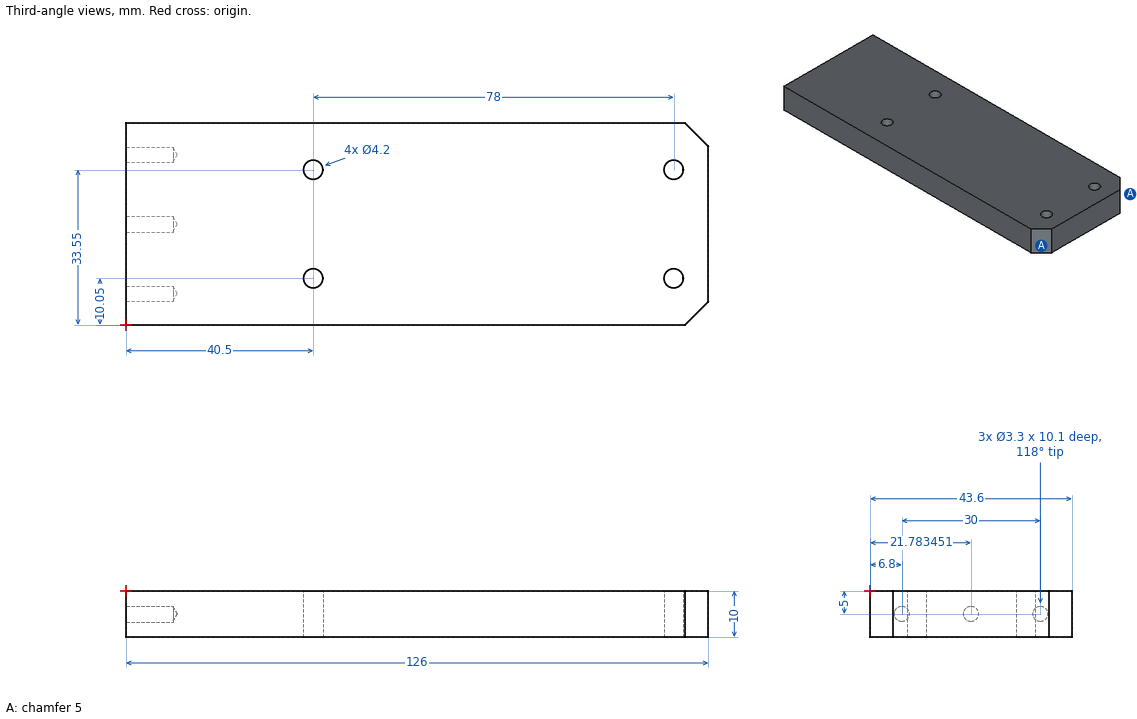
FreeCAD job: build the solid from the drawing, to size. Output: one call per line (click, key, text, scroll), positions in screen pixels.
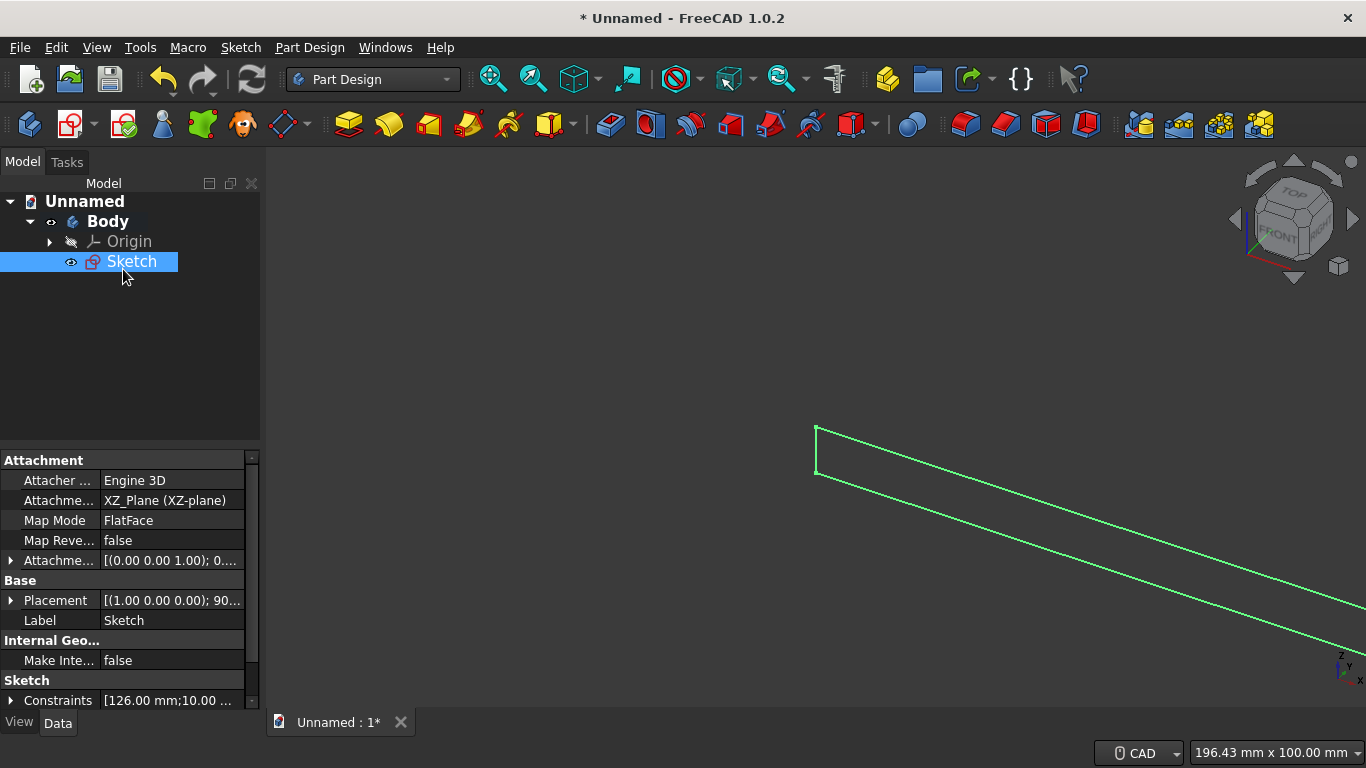
click(350, 124)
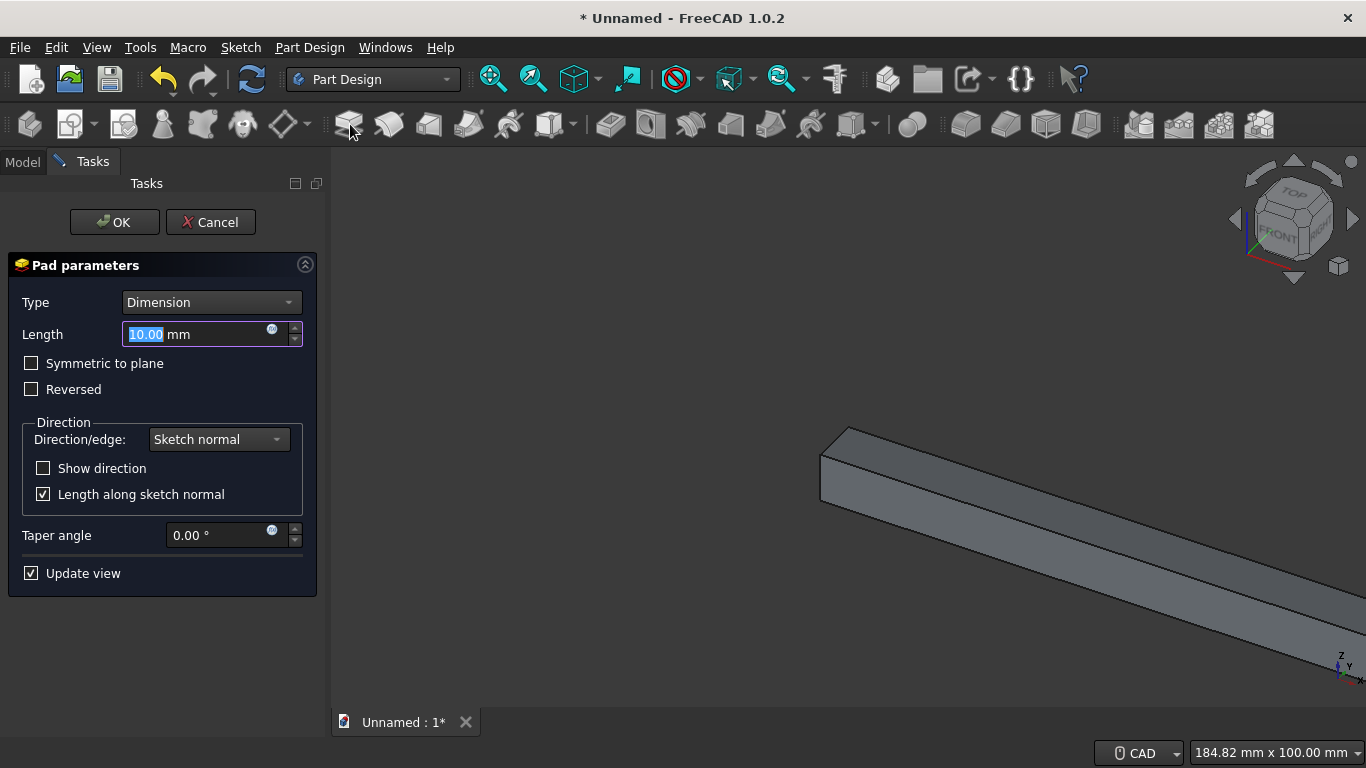
text(43.6)
key(Tab)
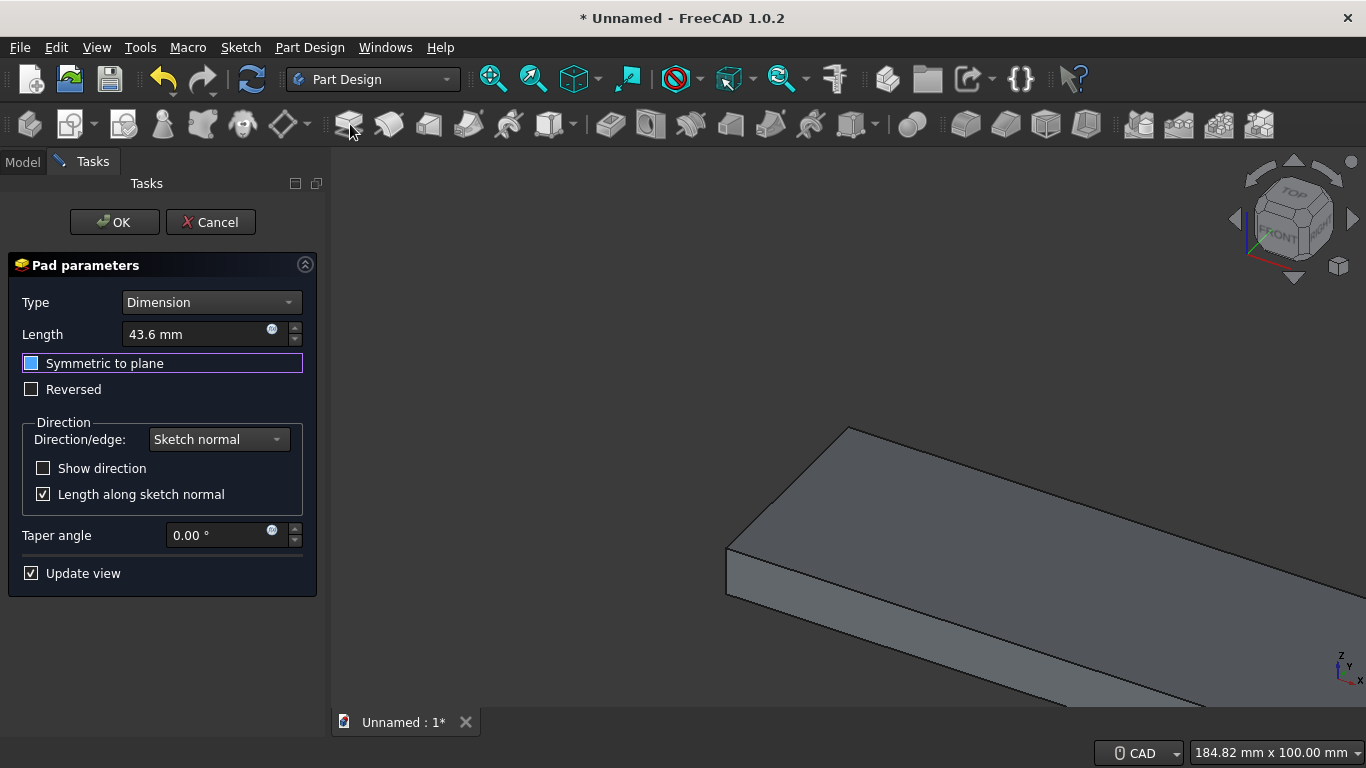
click(30, 389)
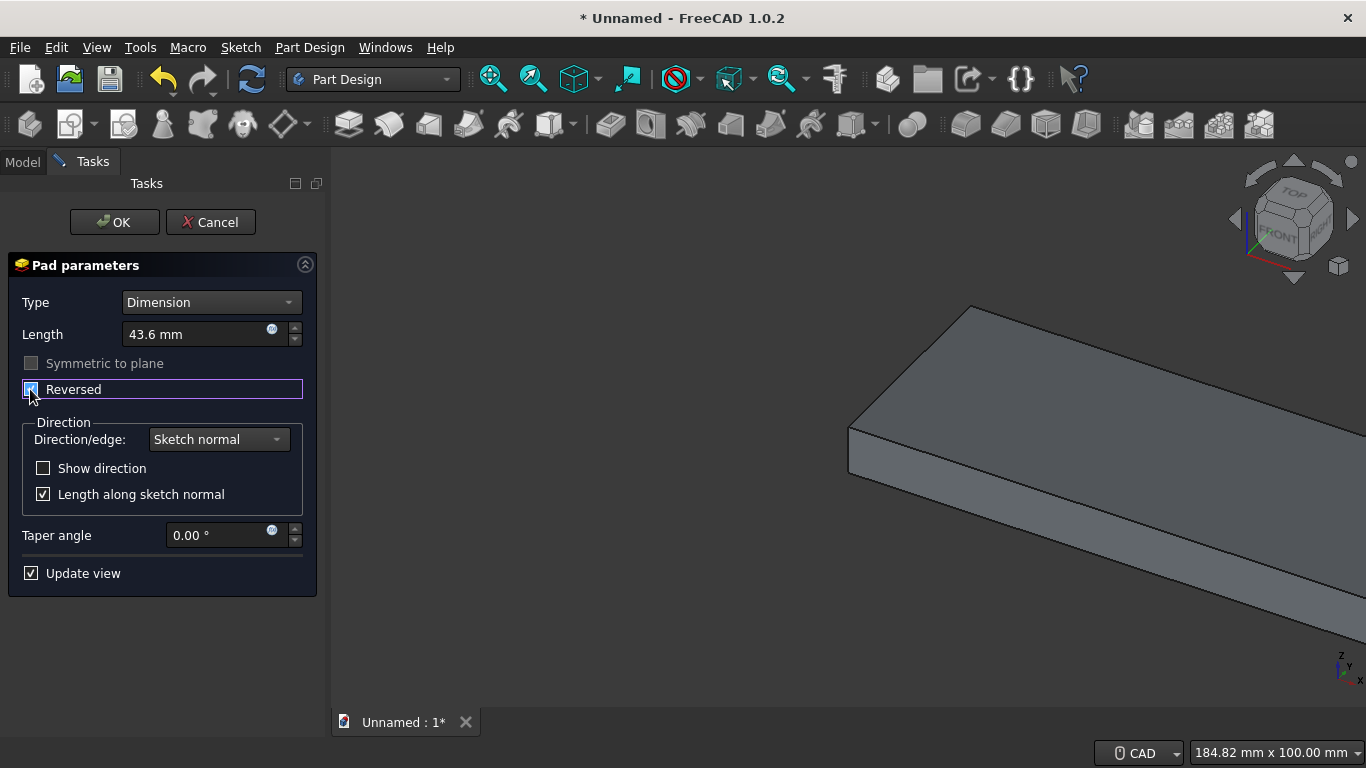
click(115, 222)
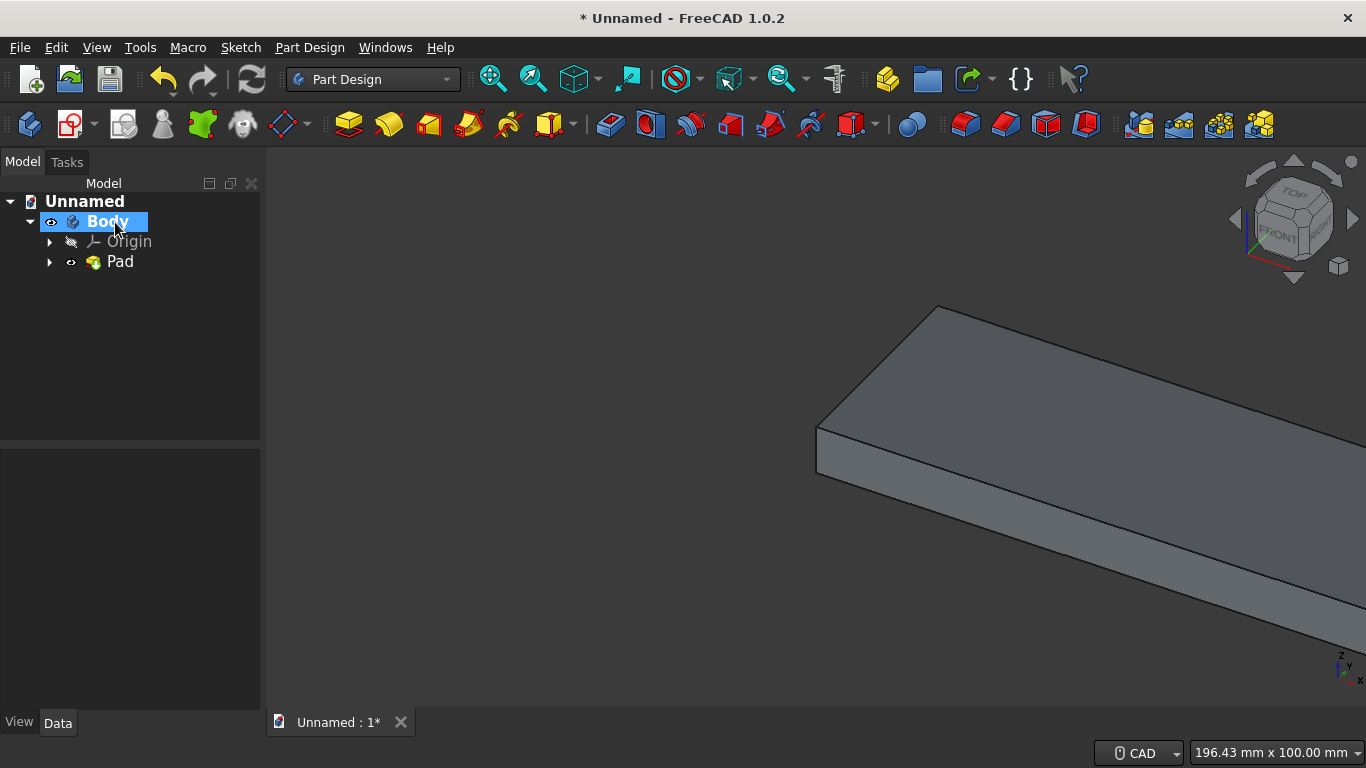
click(494, 80)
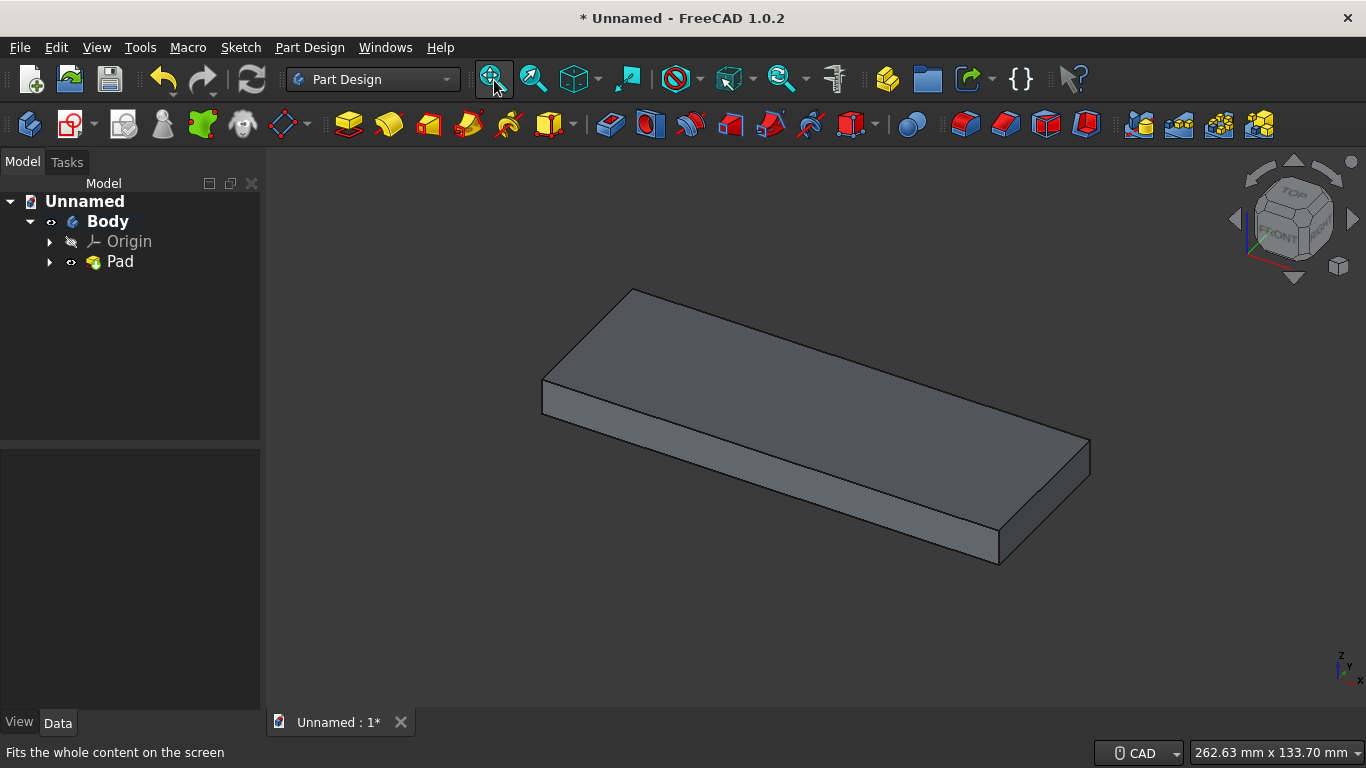
click(999, 547)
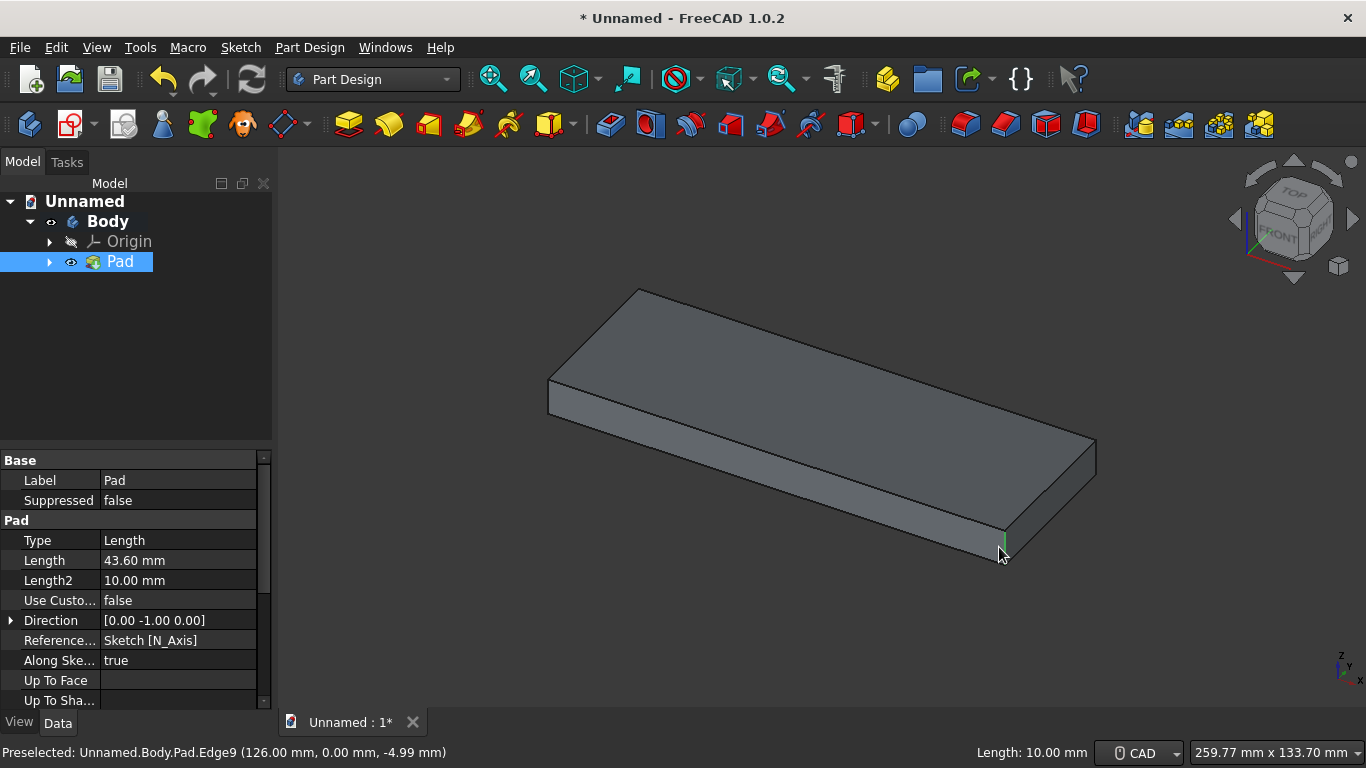
key(0)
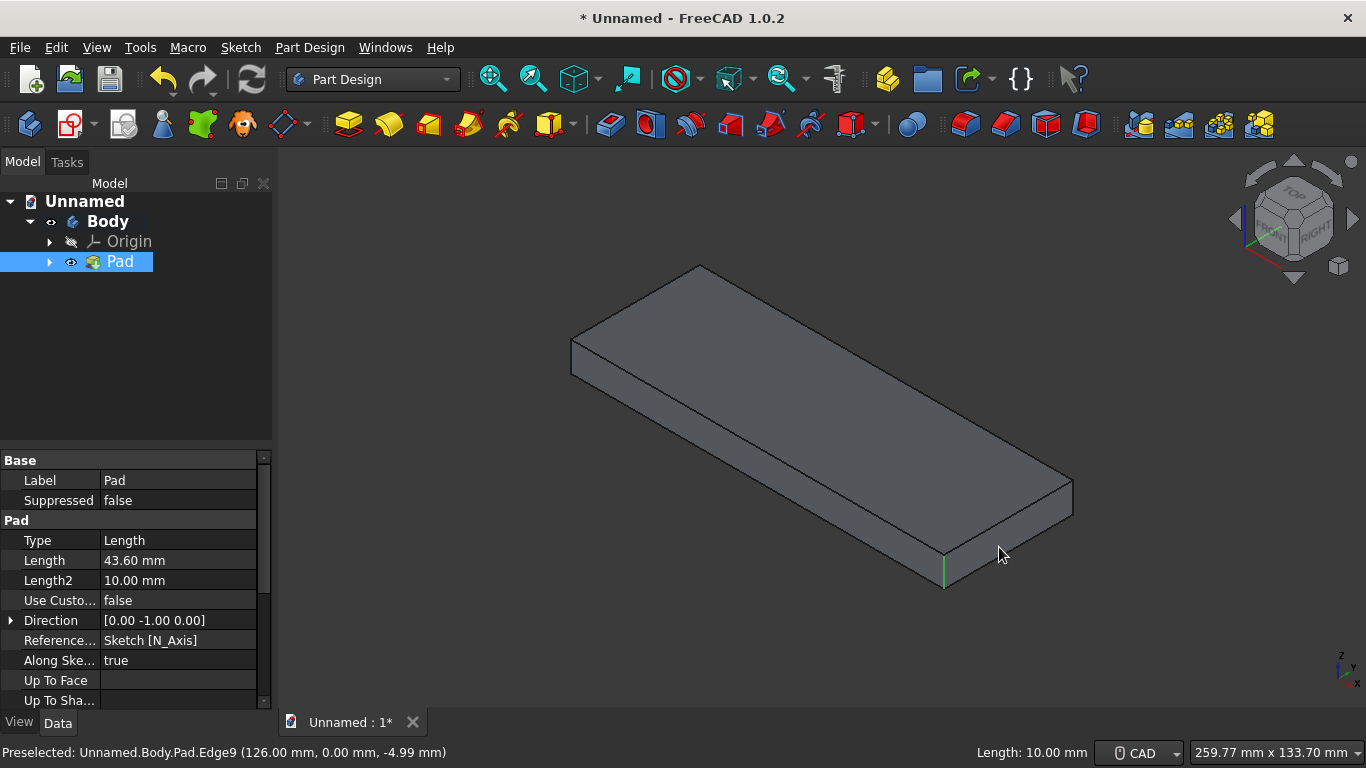
key(2)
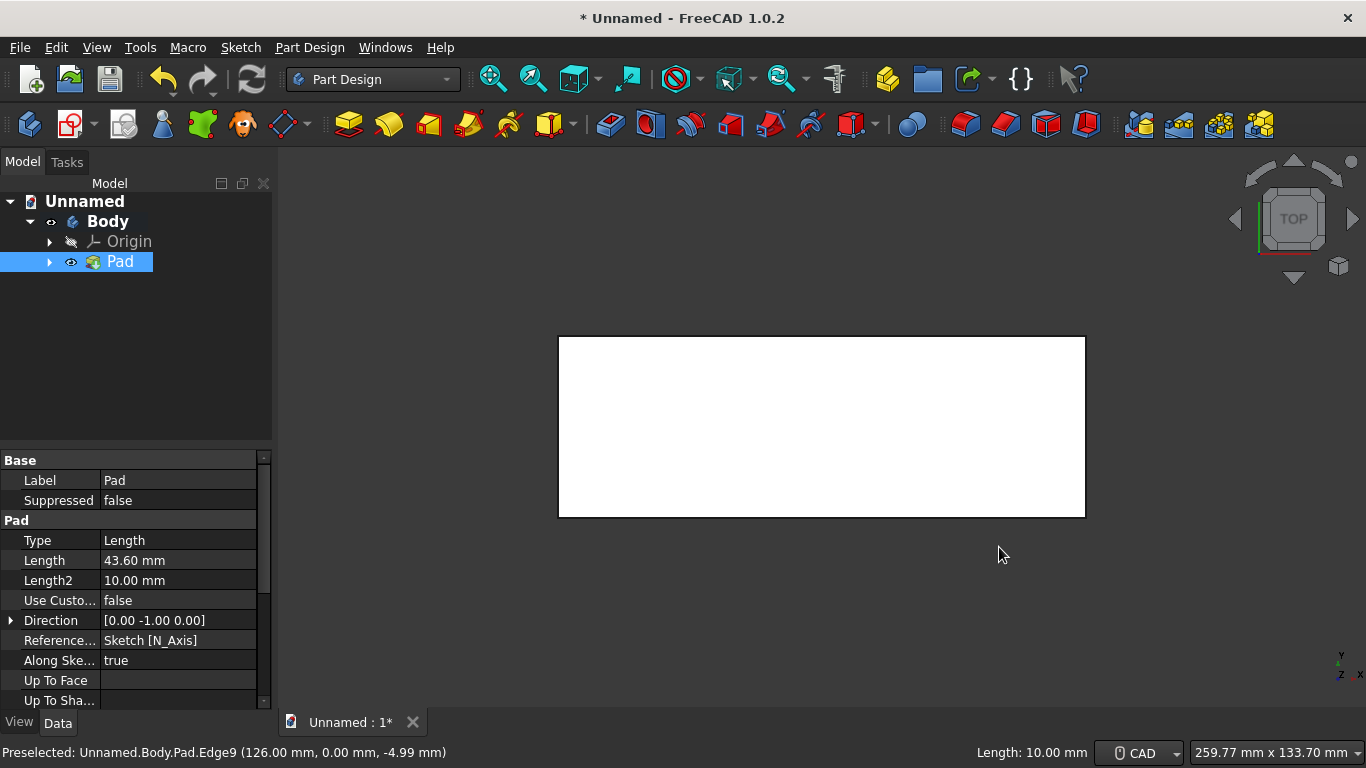
key(1)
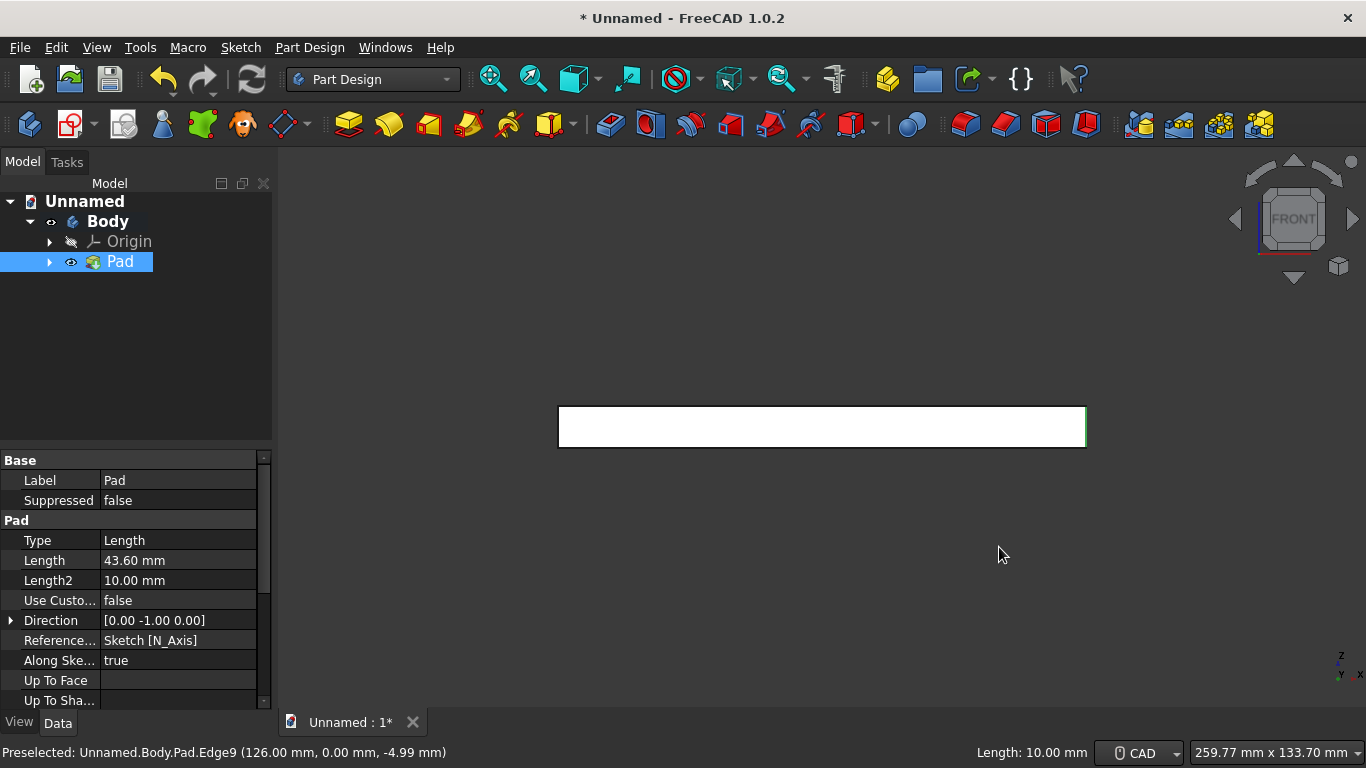
key(3)